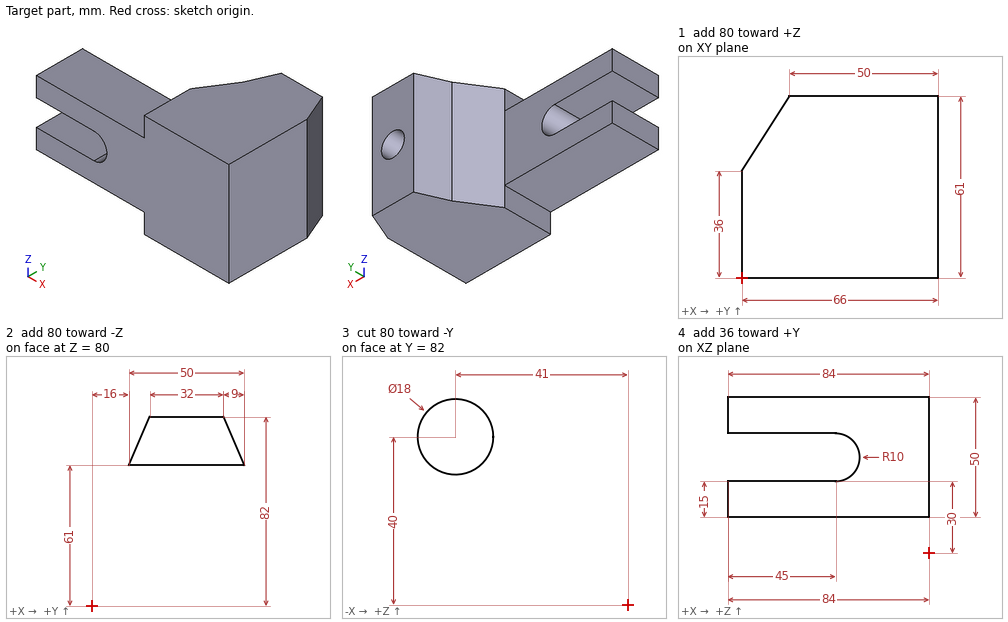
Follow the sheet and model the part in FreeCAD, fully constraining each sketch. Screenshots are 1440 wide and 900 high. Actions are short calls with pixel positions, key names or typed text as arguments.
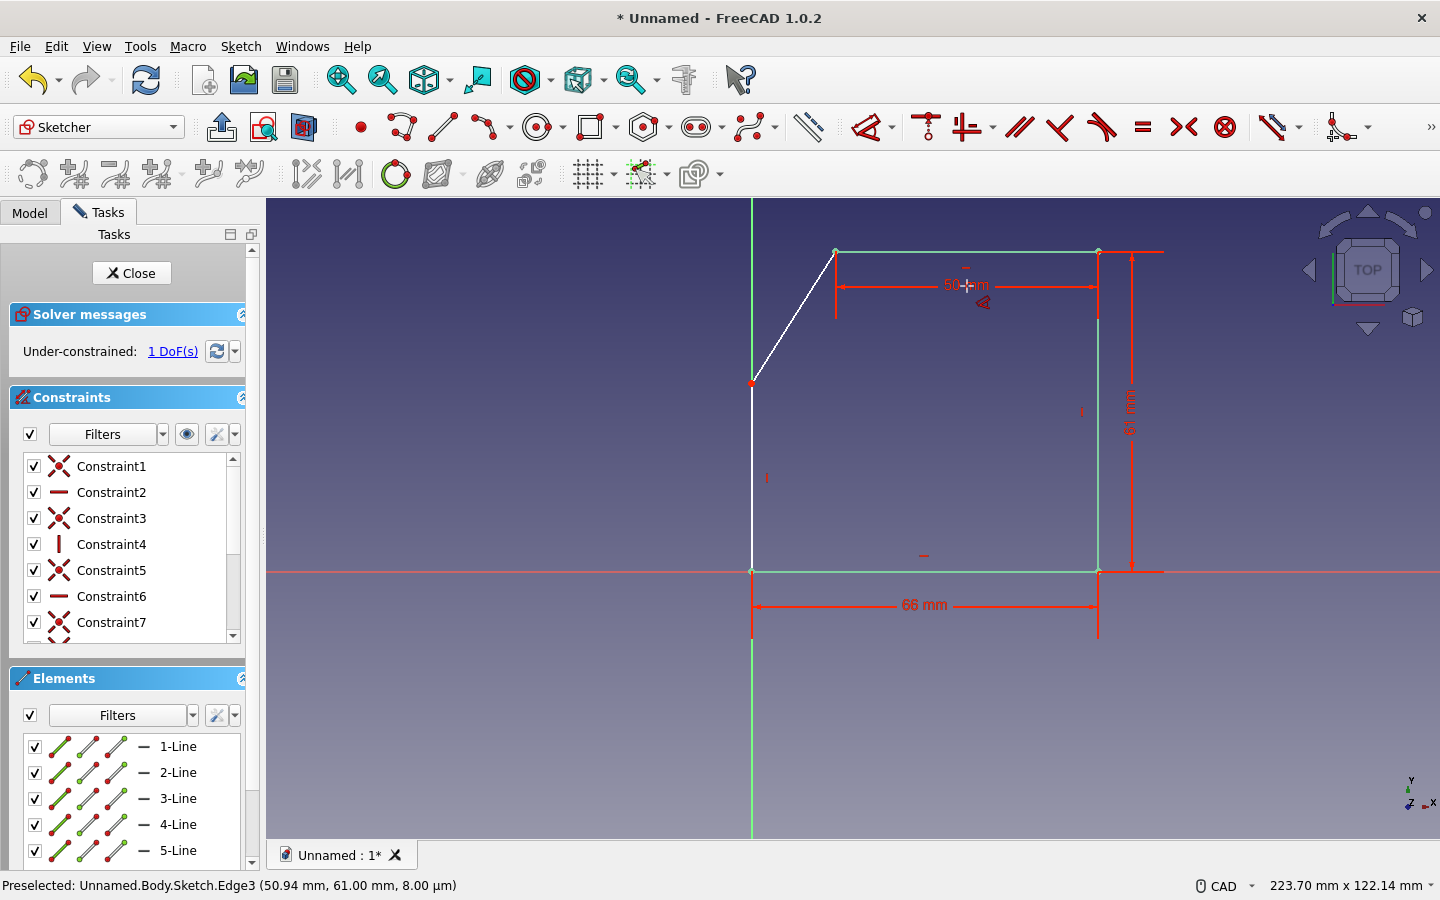
click(752, 440)
click(718, 478)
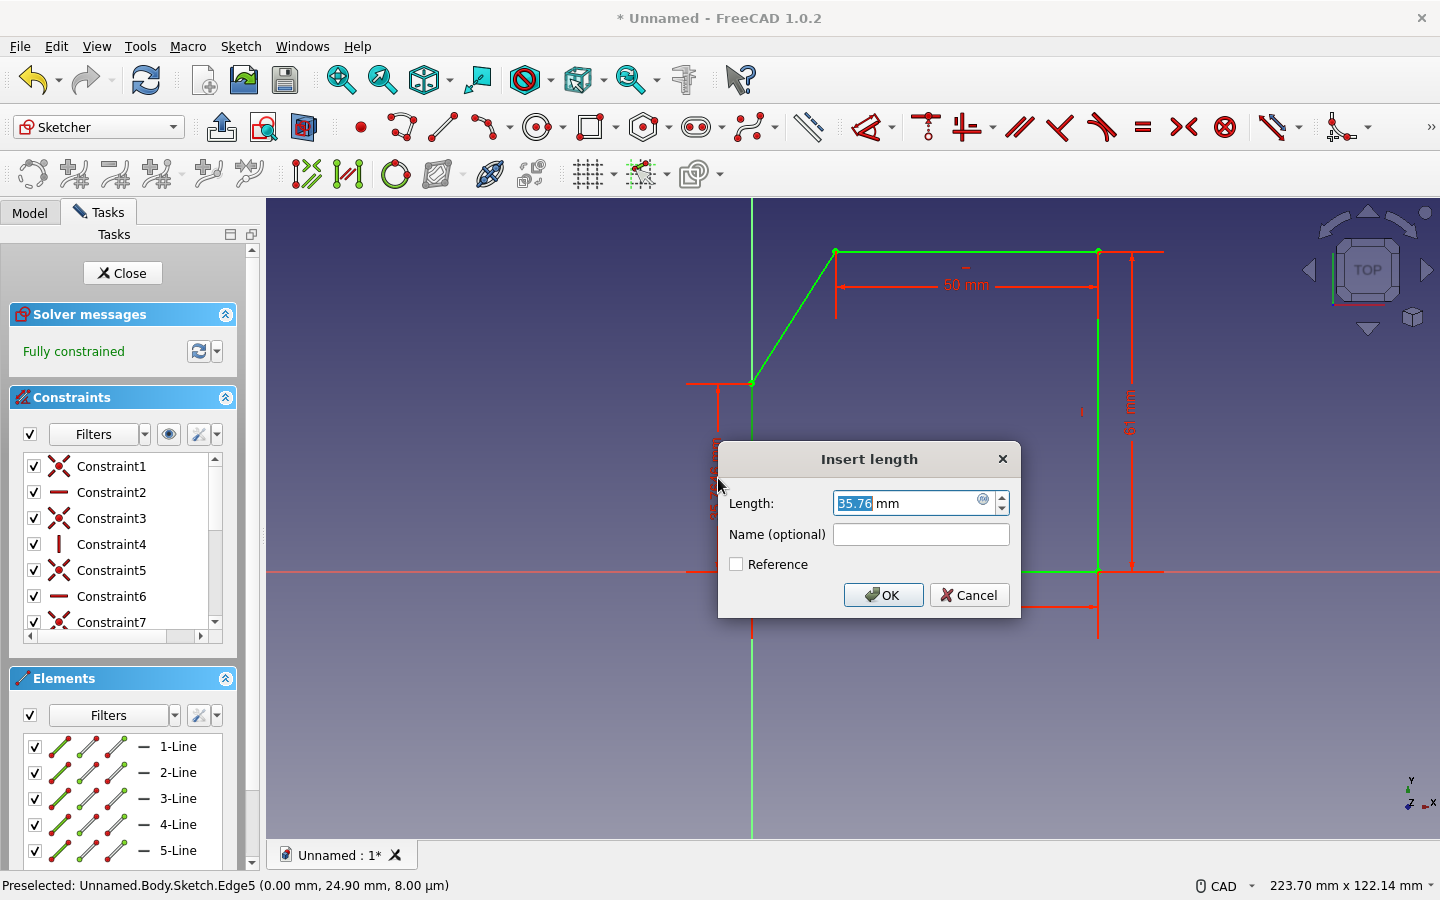
text(36)
key(Return)
key(Escape)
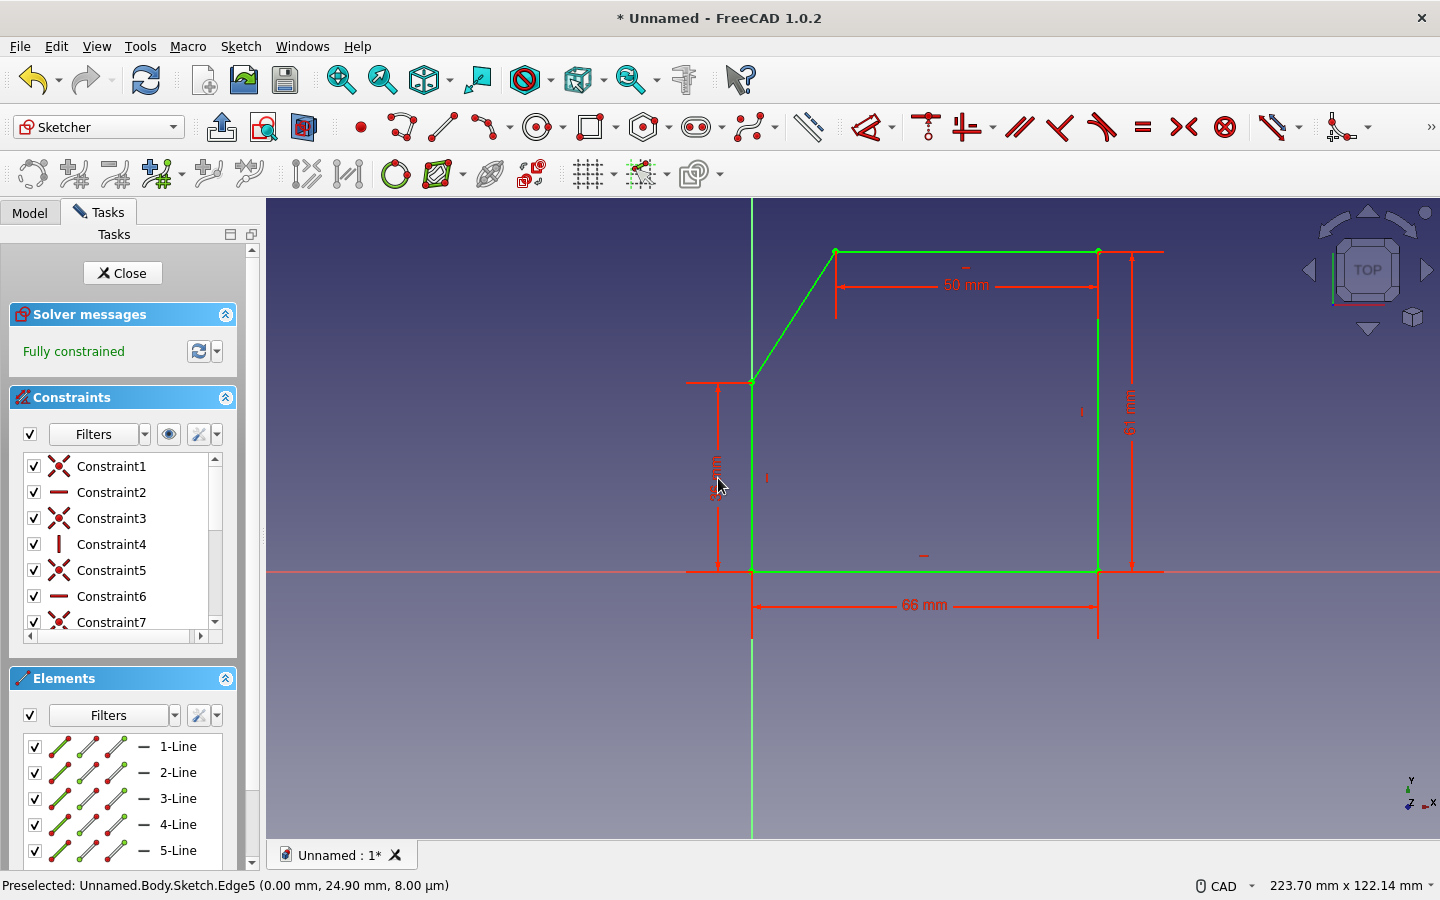
click(123, 273)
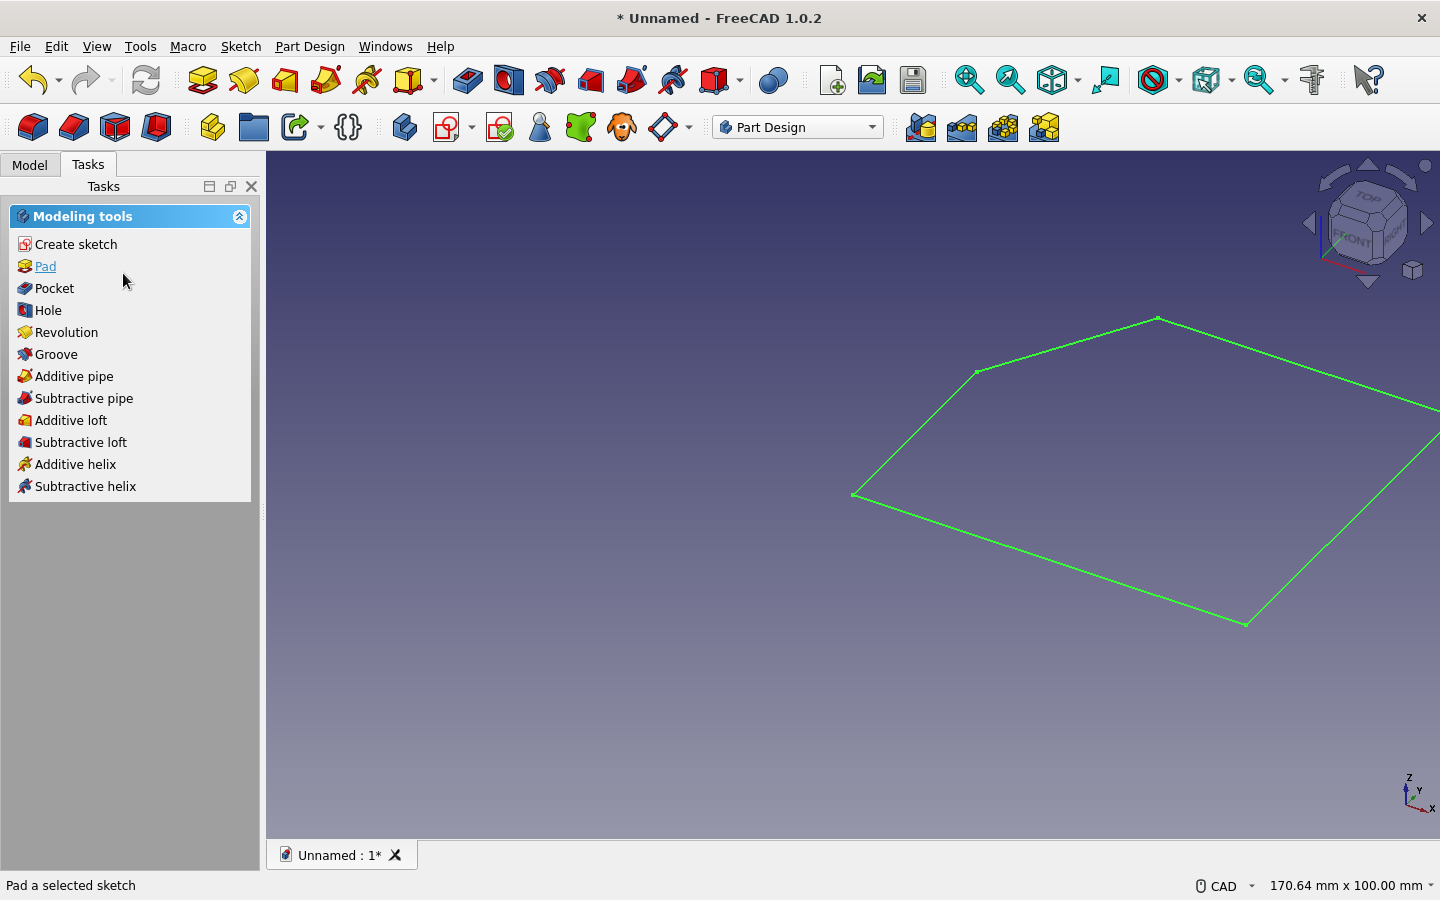
click(203, 80)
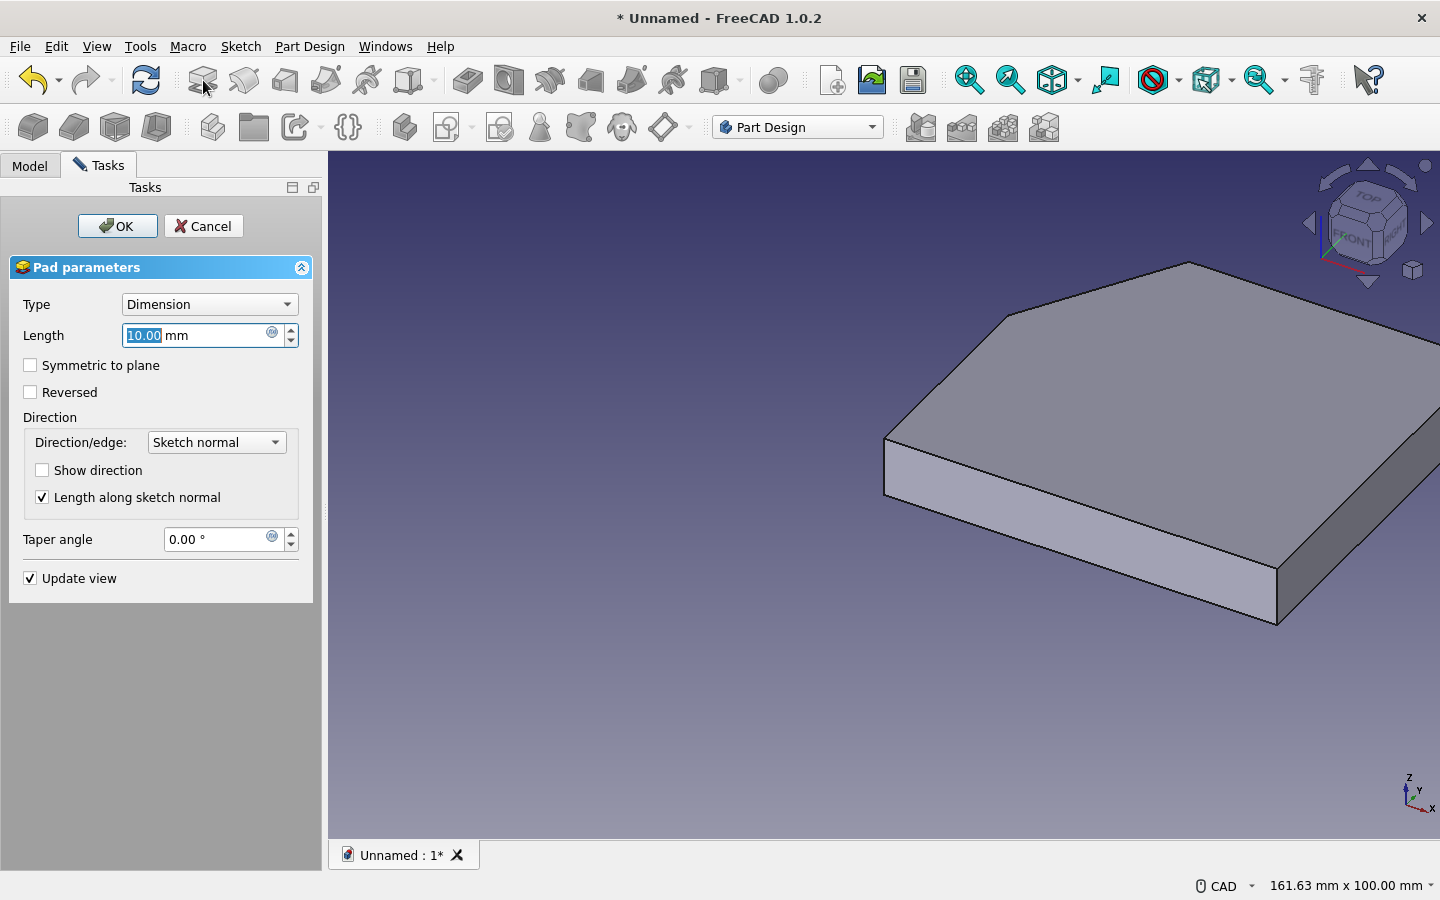
text(80)
key(Tab)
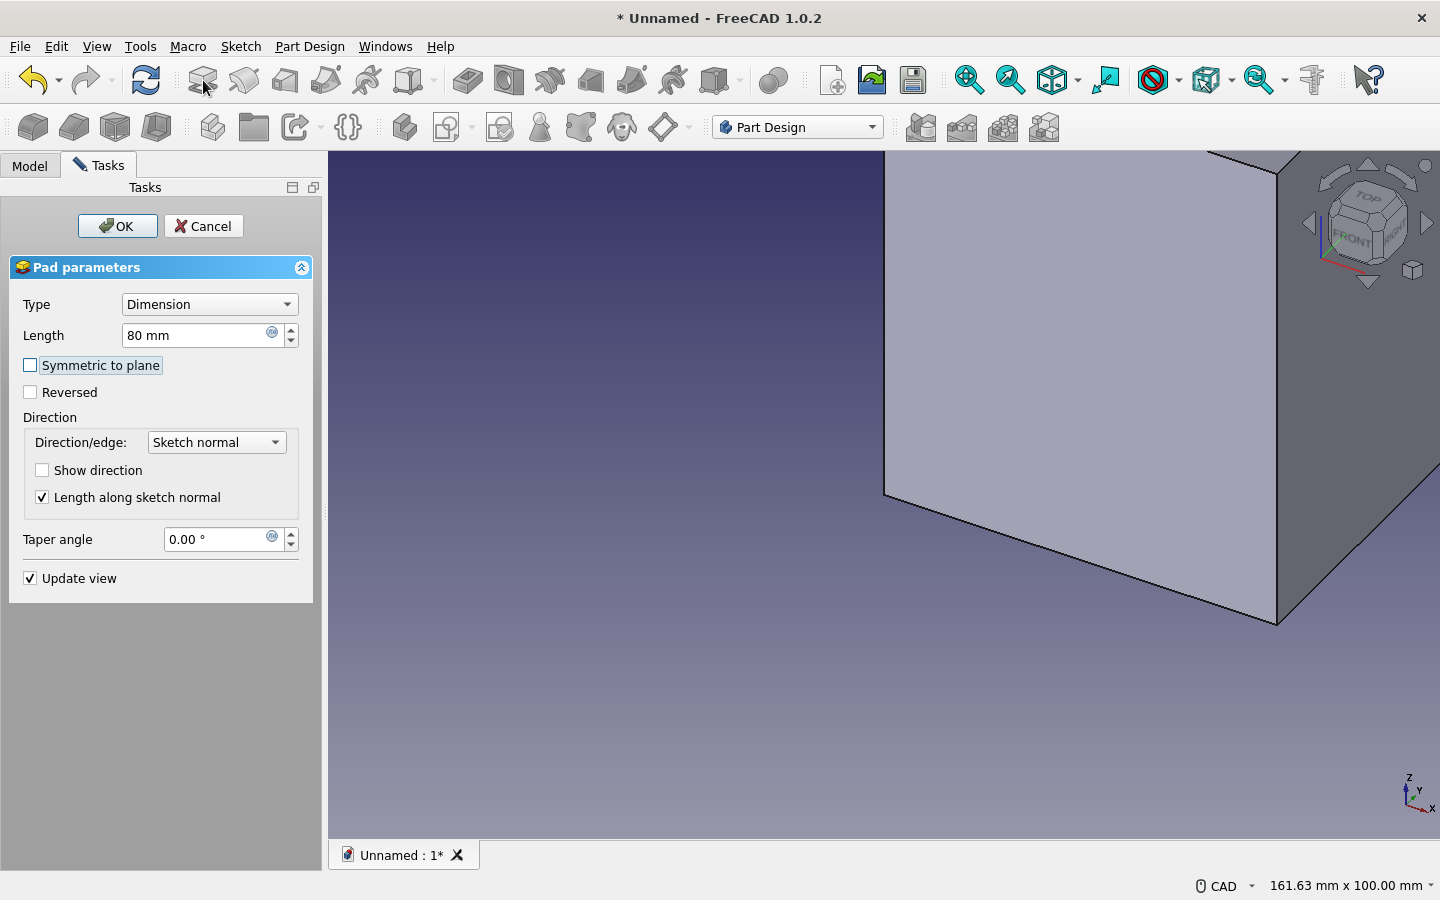
click(118, 226)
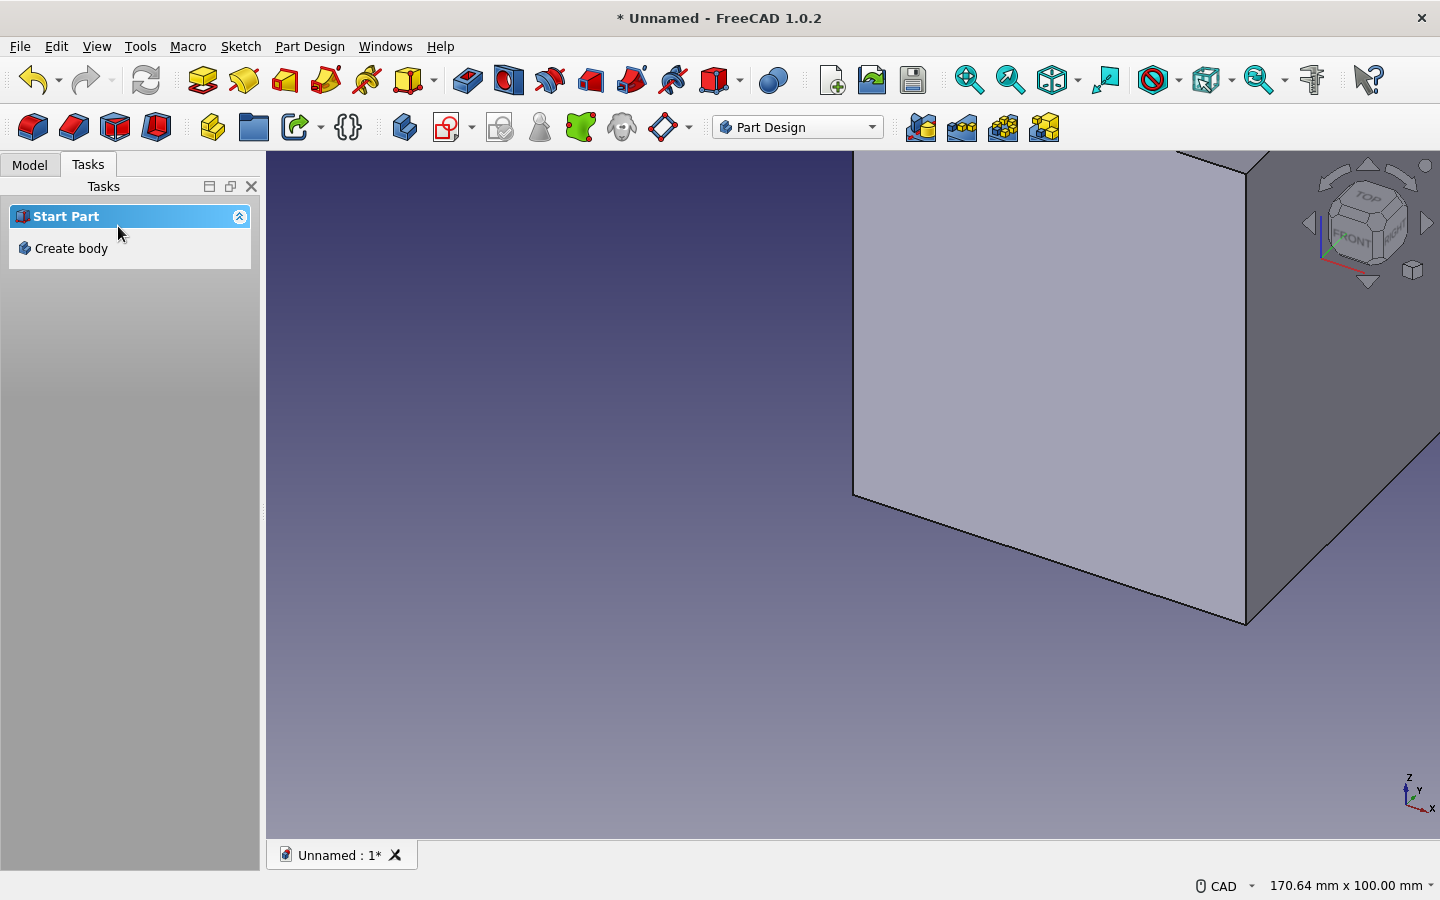
key(v)
key(f)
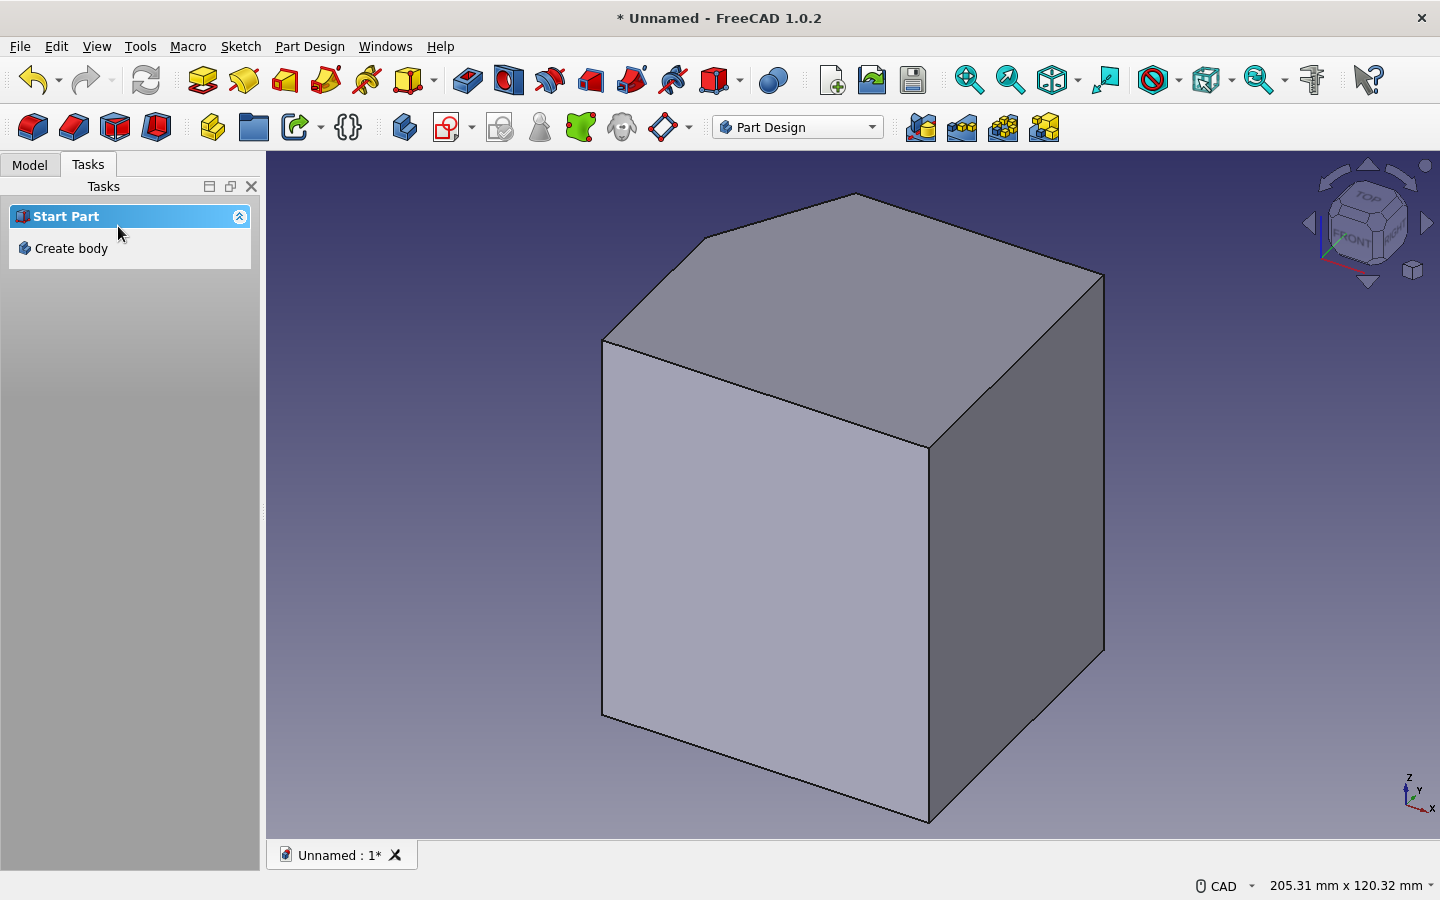
click(853, 307)